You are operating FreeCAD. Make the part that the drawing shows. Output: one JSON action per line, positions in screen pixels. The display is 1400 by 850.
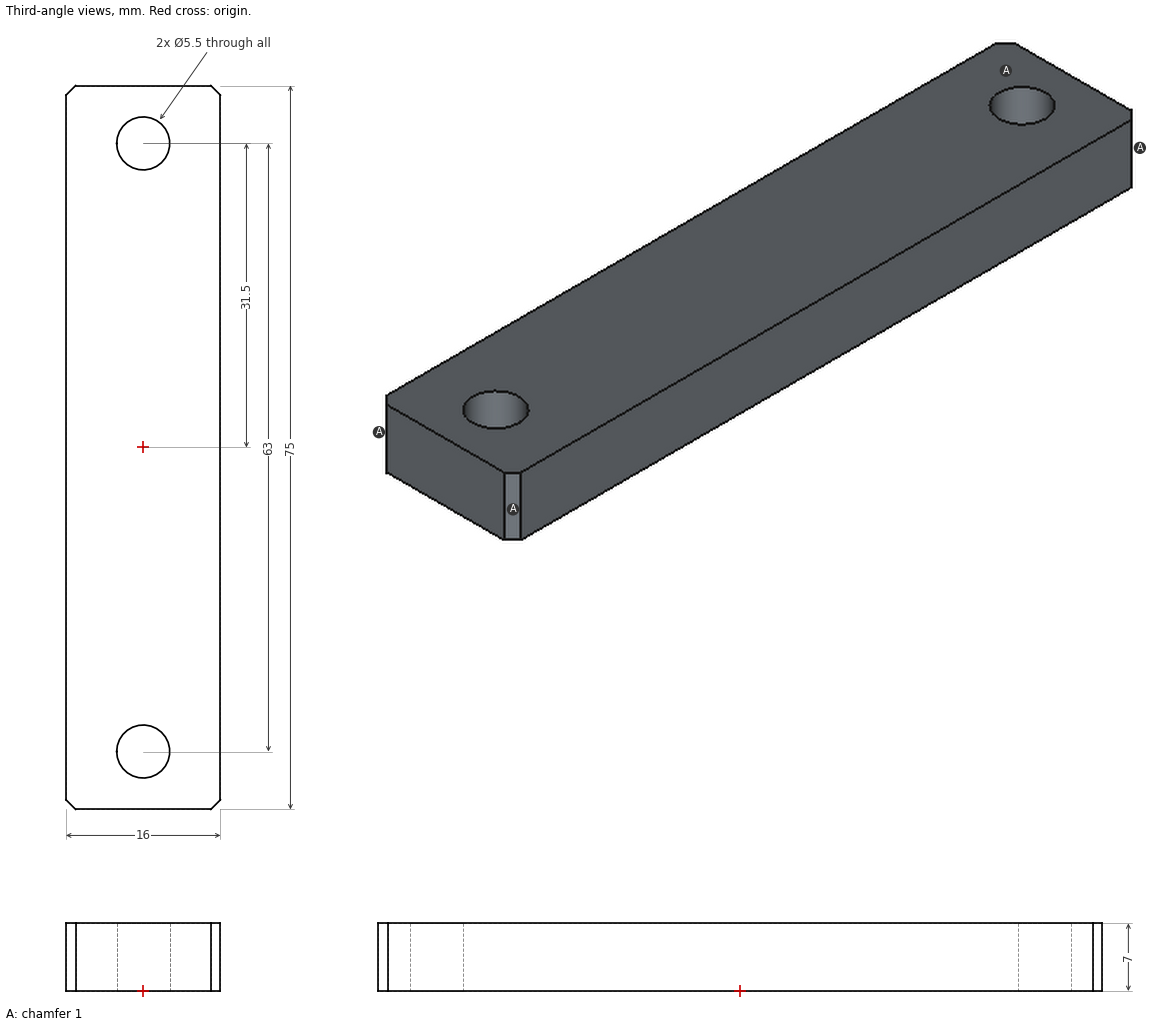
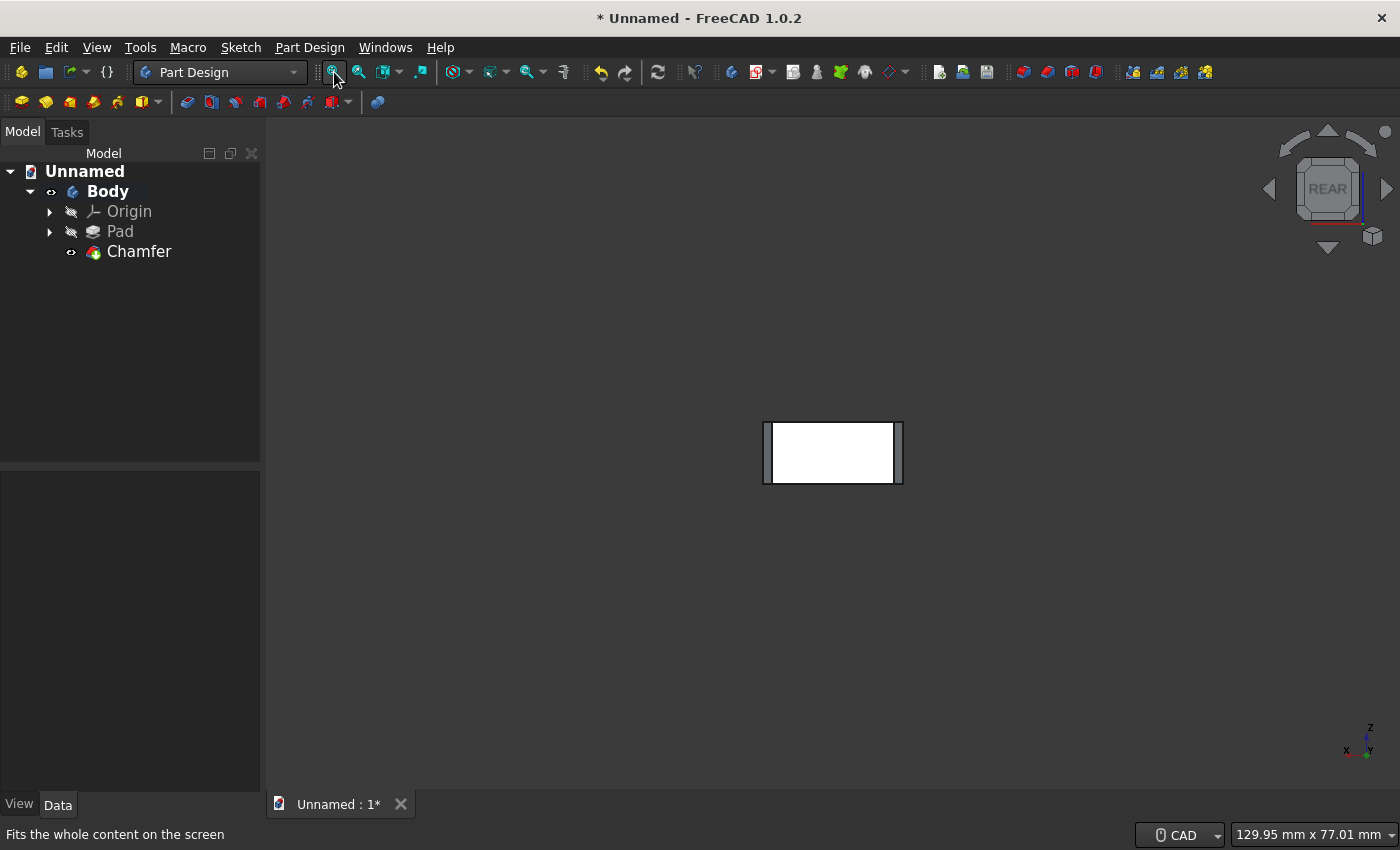
{"action": "key", "text": "0"}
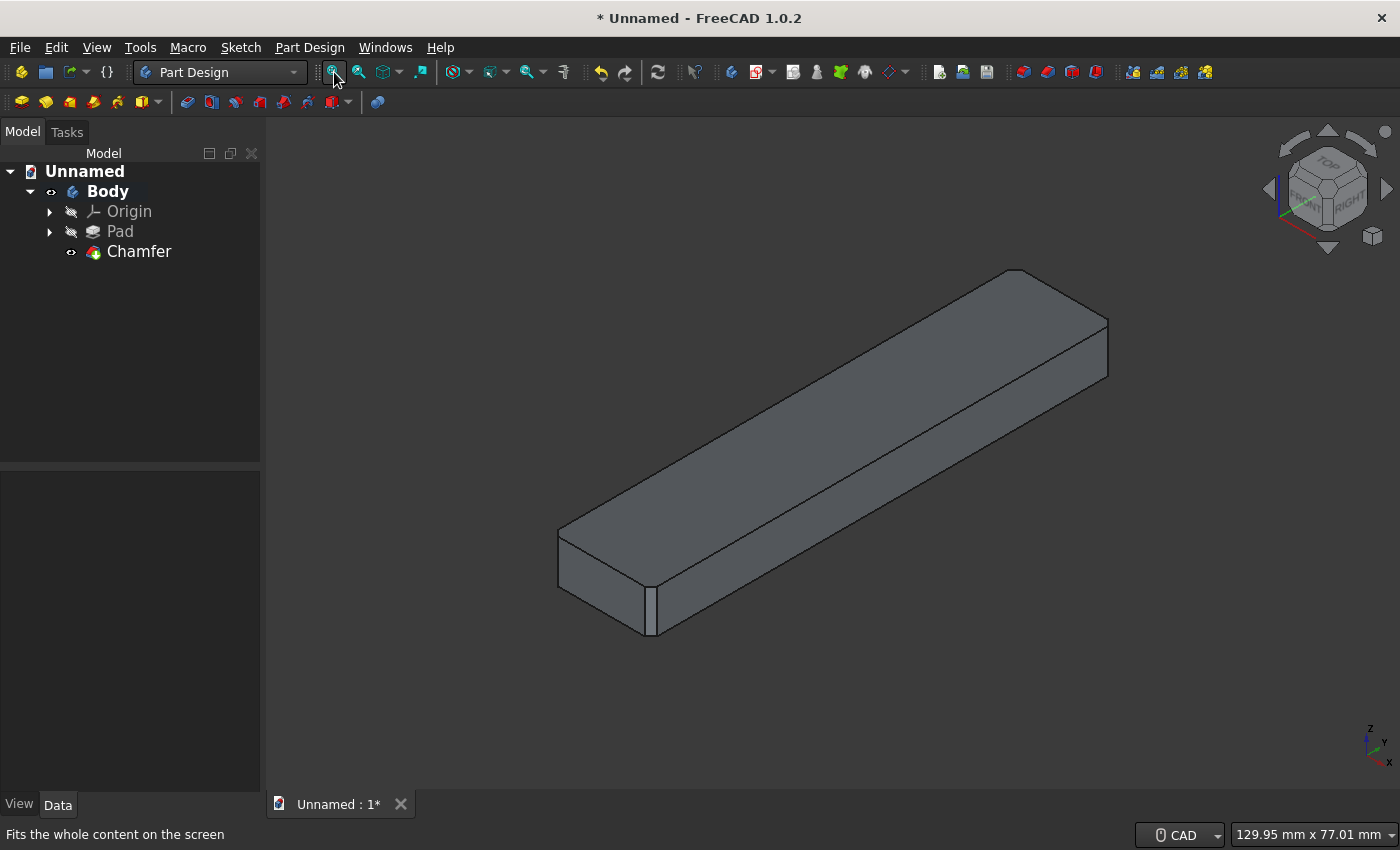
{"action": "left_click", "coordinate": [965, 351]}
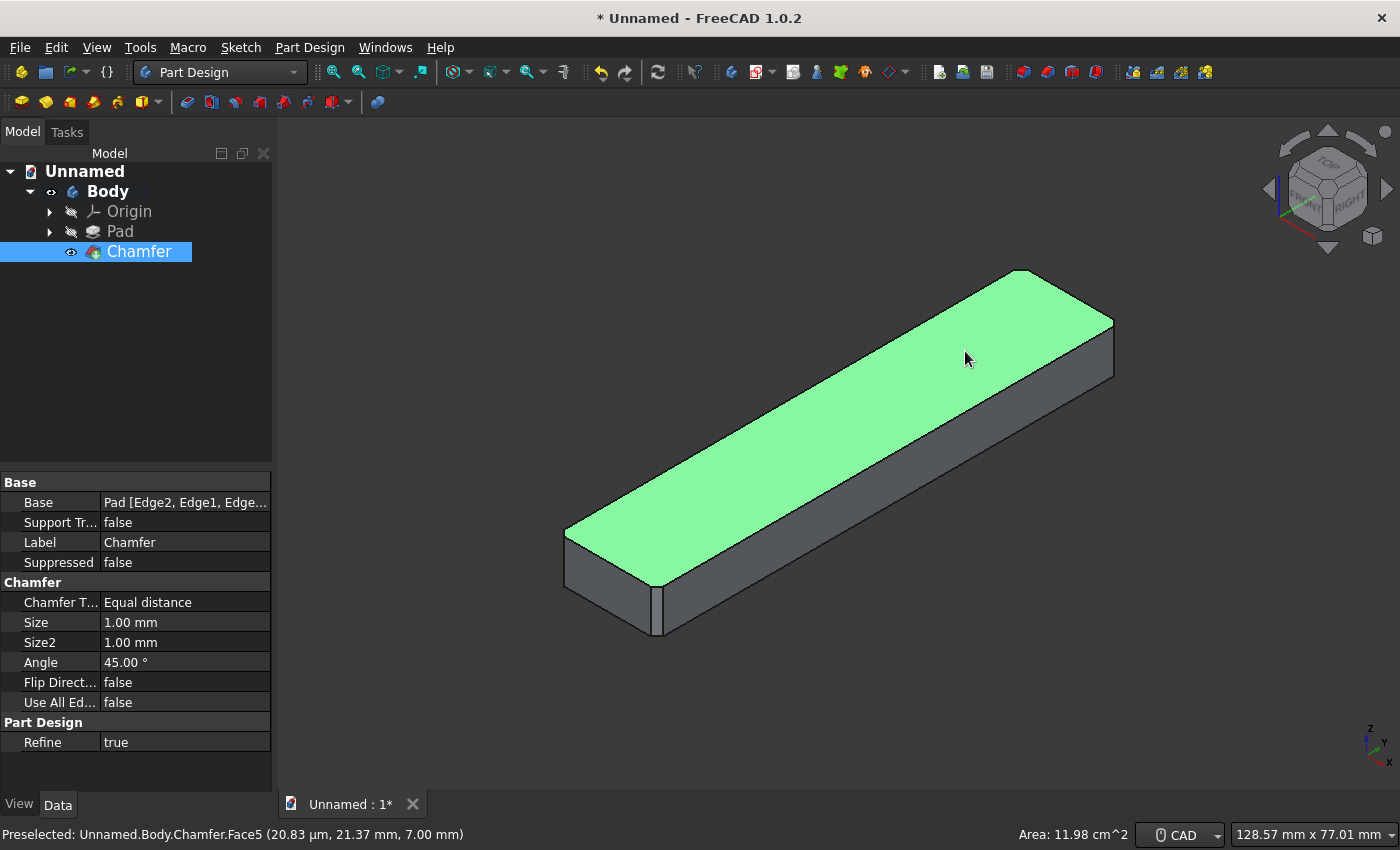
{"action": "left_click", "coordinate": [756, 72]}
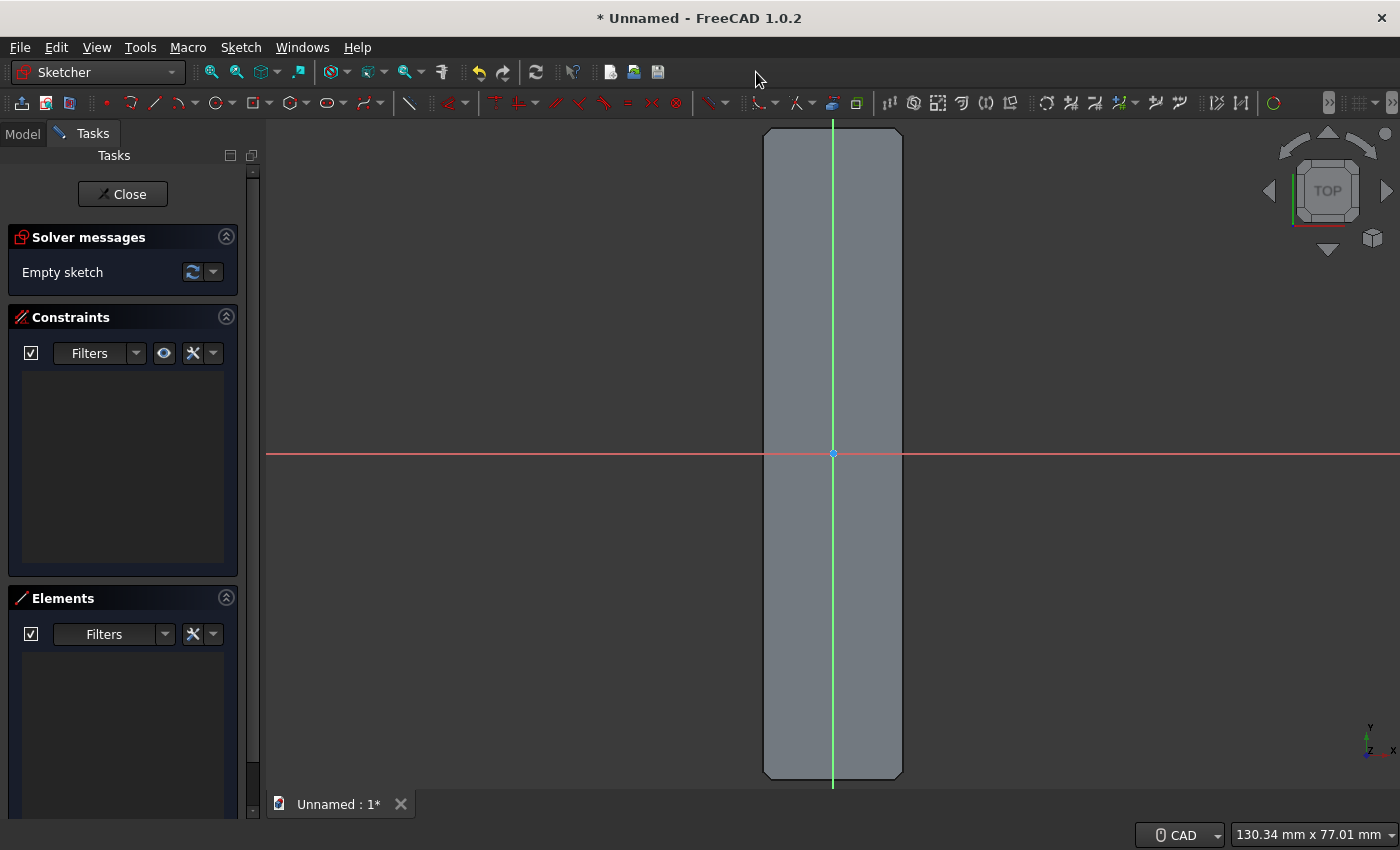
{"action": "scroll", "coordinate": [625, 454], "scroll_direction": "down", "scroll_amount": 2}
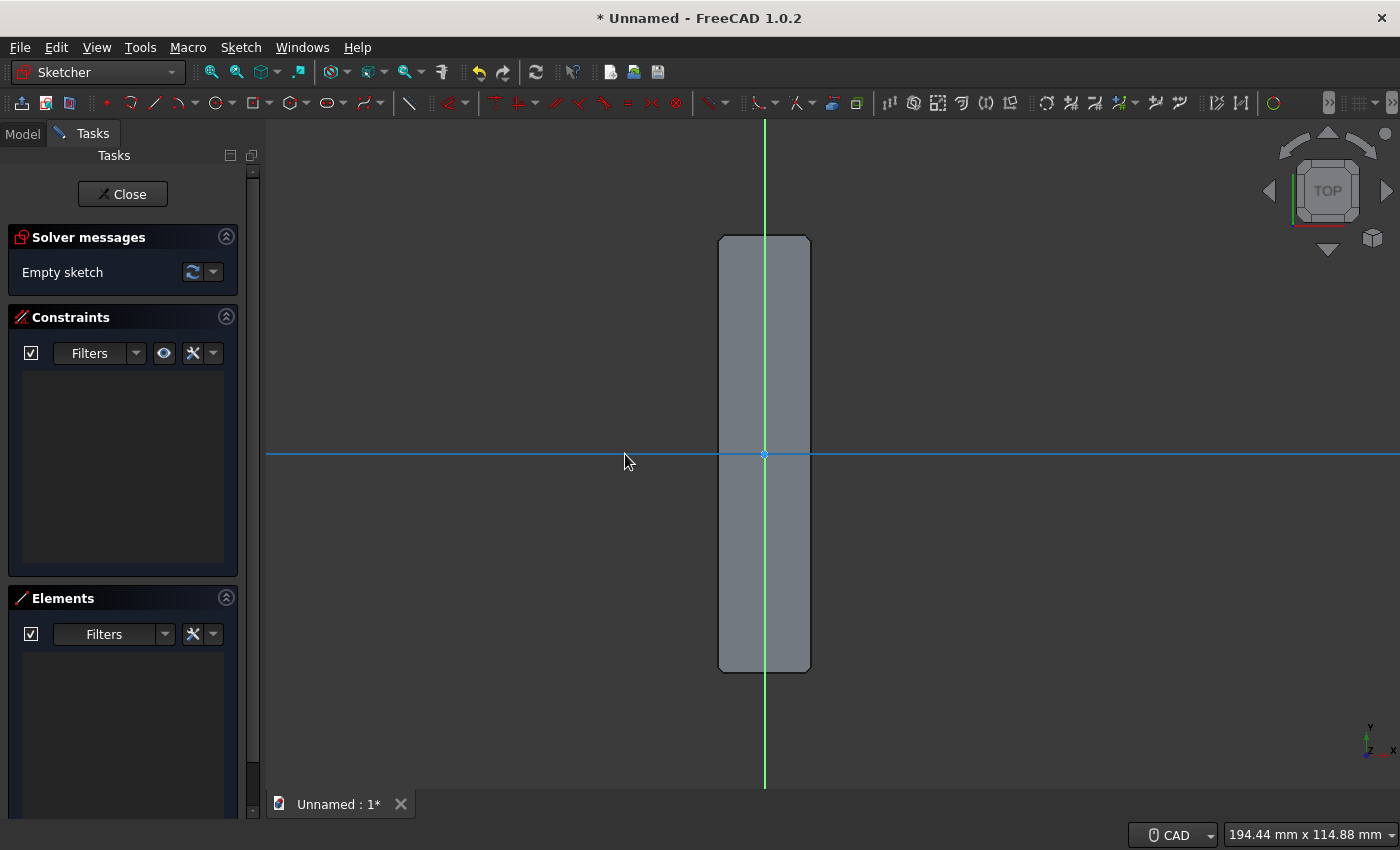
{"action": "left_click", "coordinate": [216, 104]}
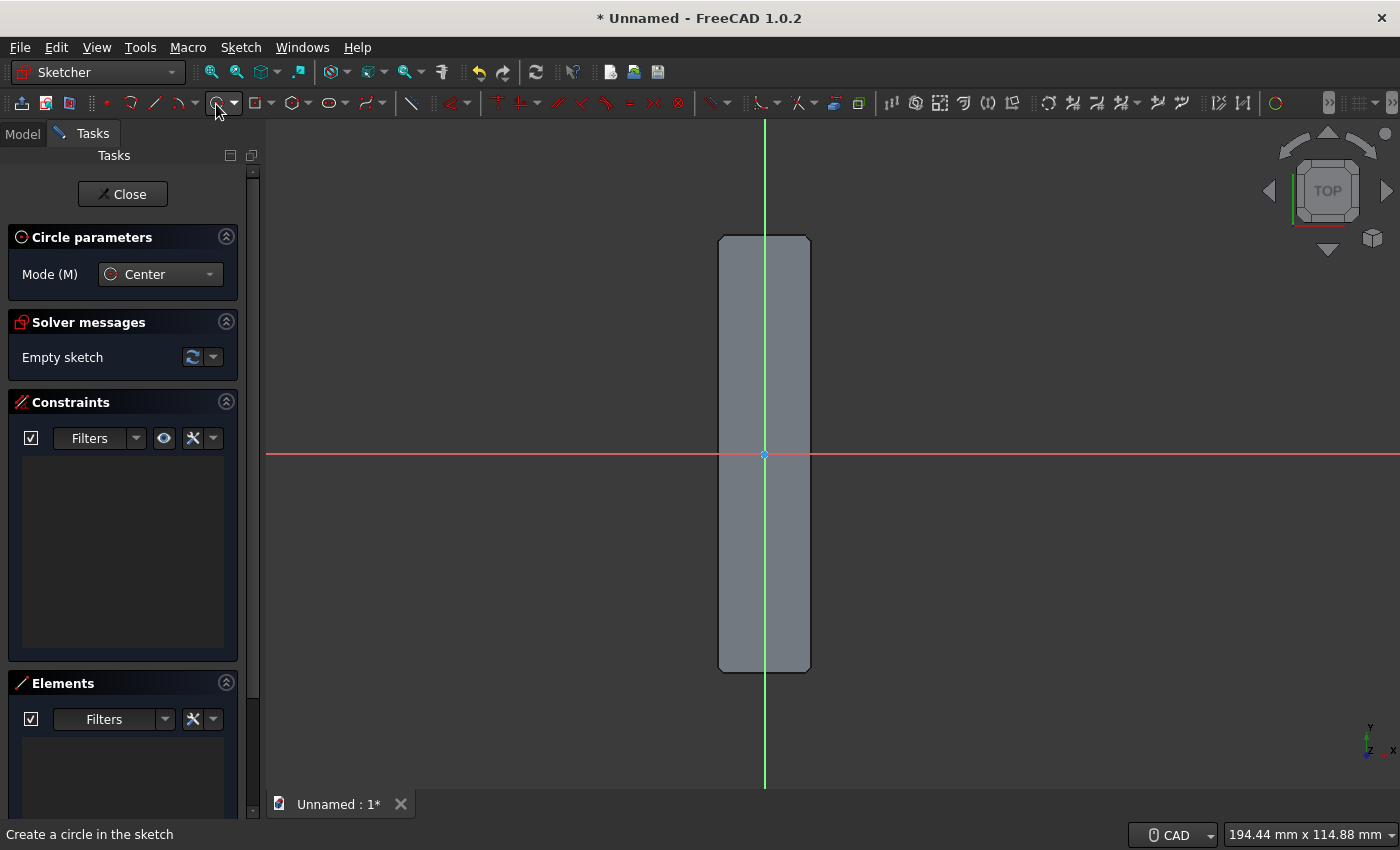
{"action": "scroll", "coordinate": [765, 270], "scroll_direction": "up", "scroll_amount": 2}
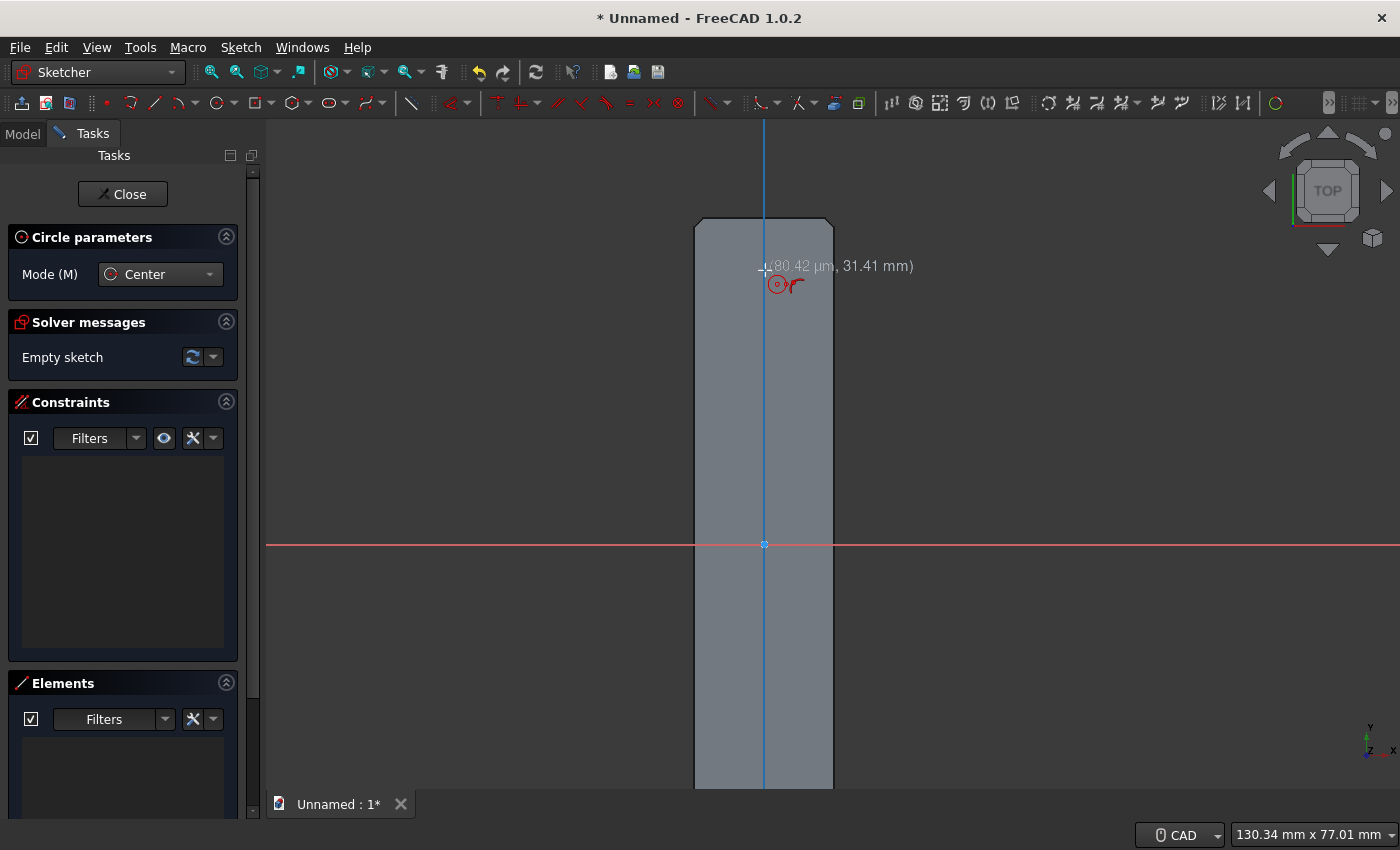
{"action": "left_click", "coordinate": [764, 271]}
{"action": "left_click", "coordinate": [781, 254]}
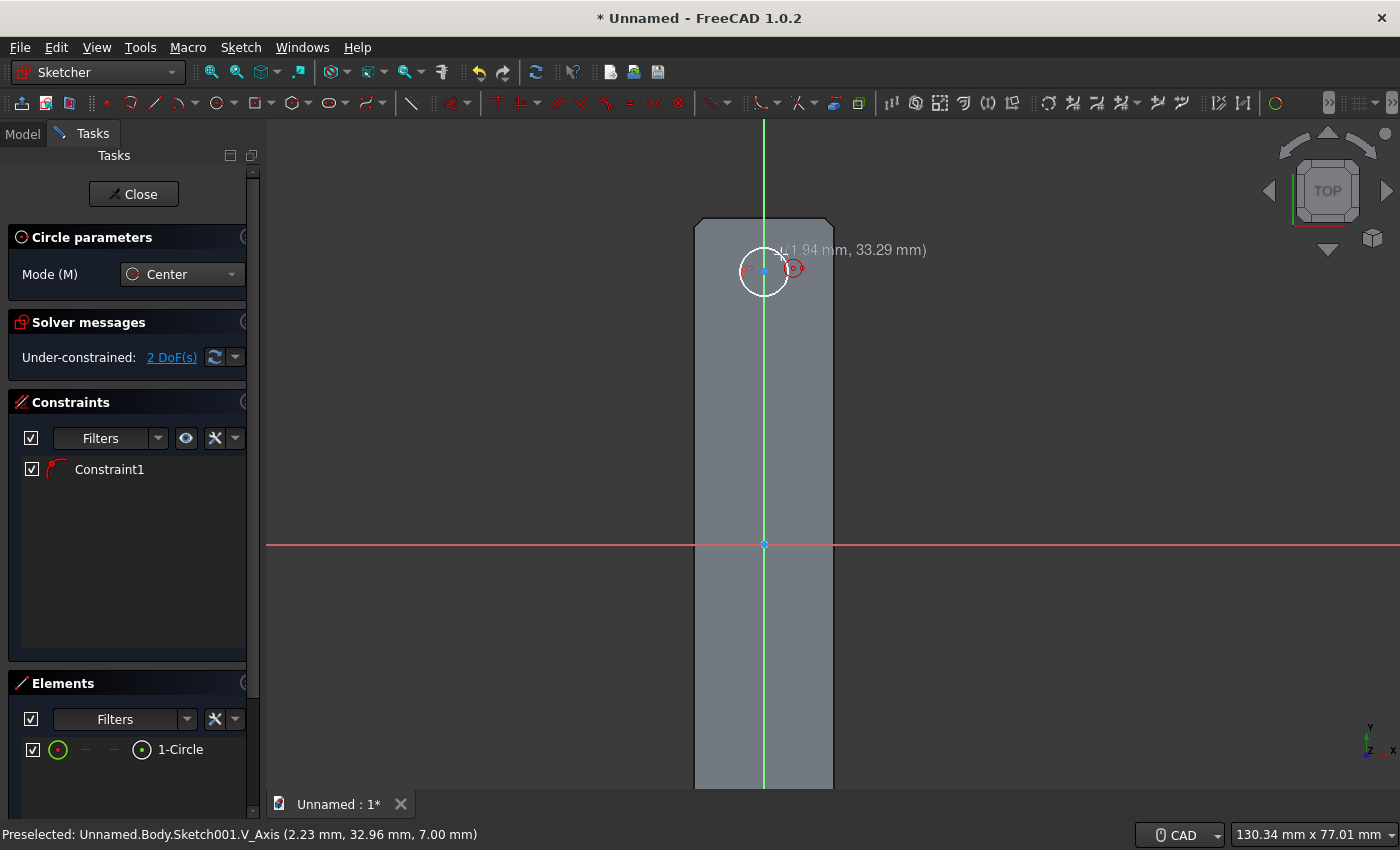
{"action": "scroll", "coordinate": [765, 270], "scroll_direction": "down", "scroll_amount": 2}